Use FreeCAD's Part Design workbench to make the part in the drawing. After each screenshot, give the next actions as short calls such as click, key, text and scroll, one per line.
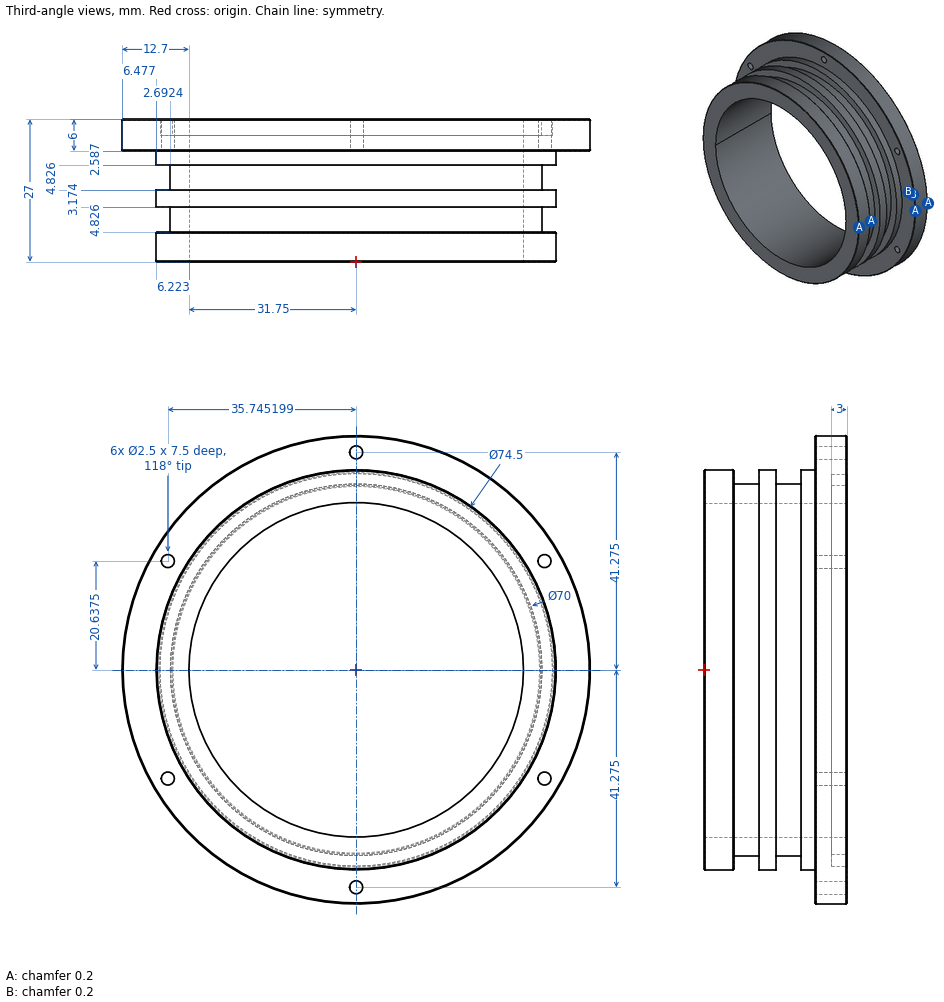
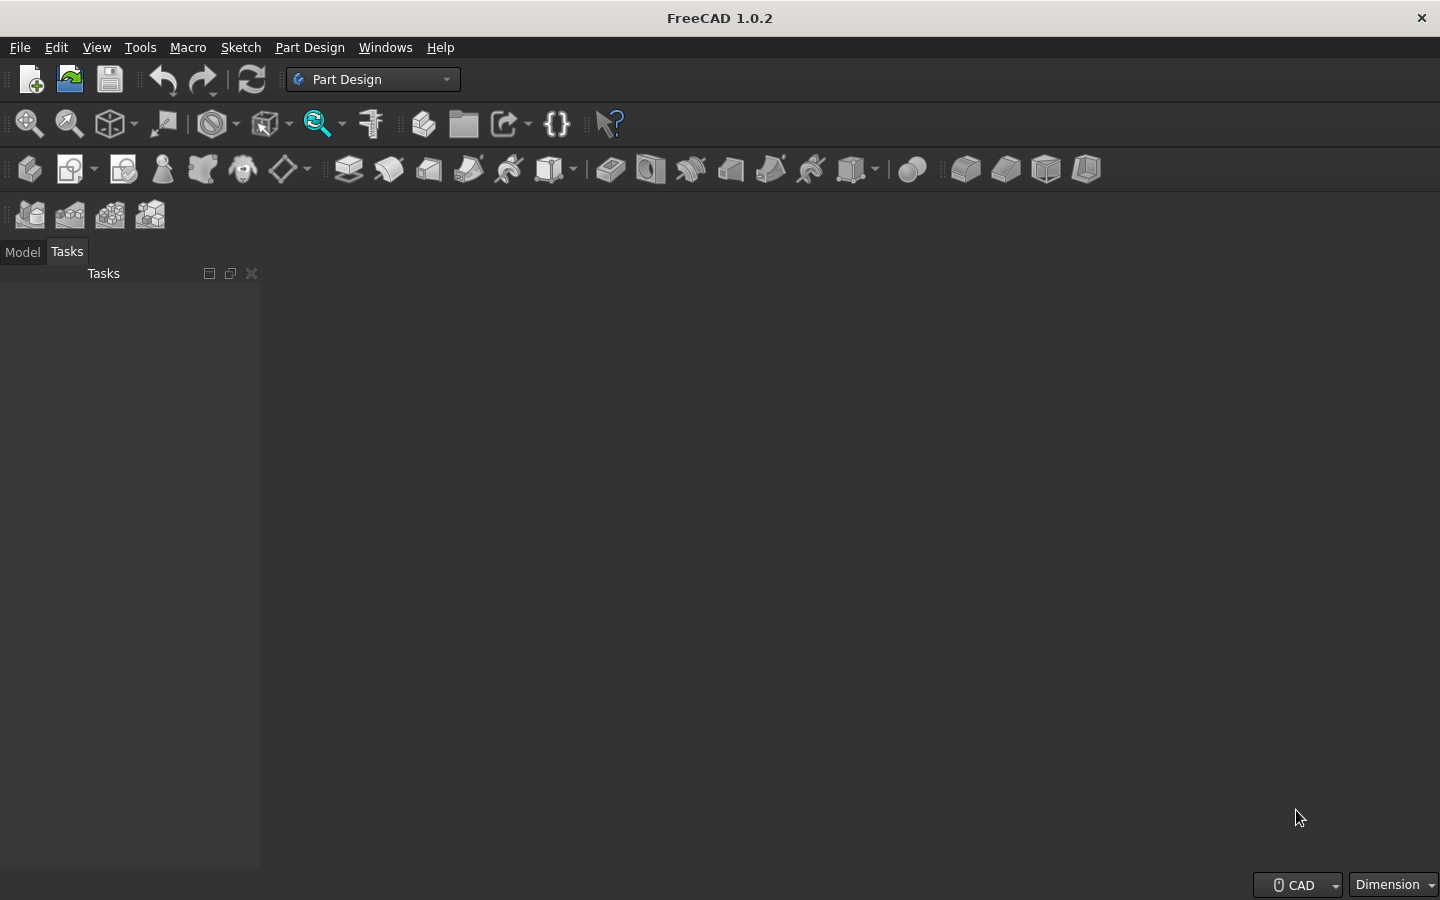
click(30, 80)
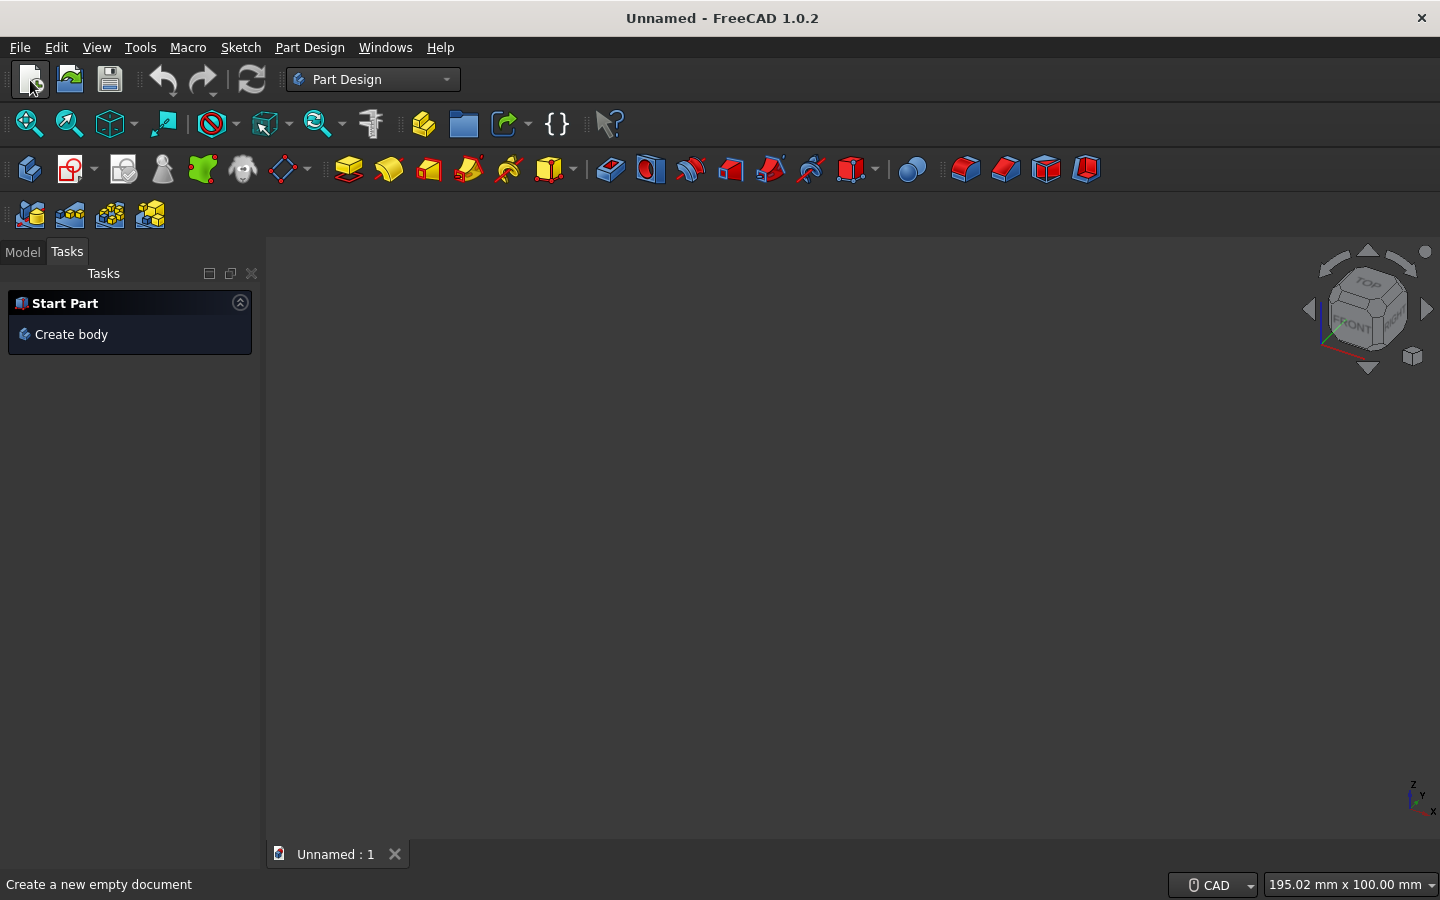
click(70, 170)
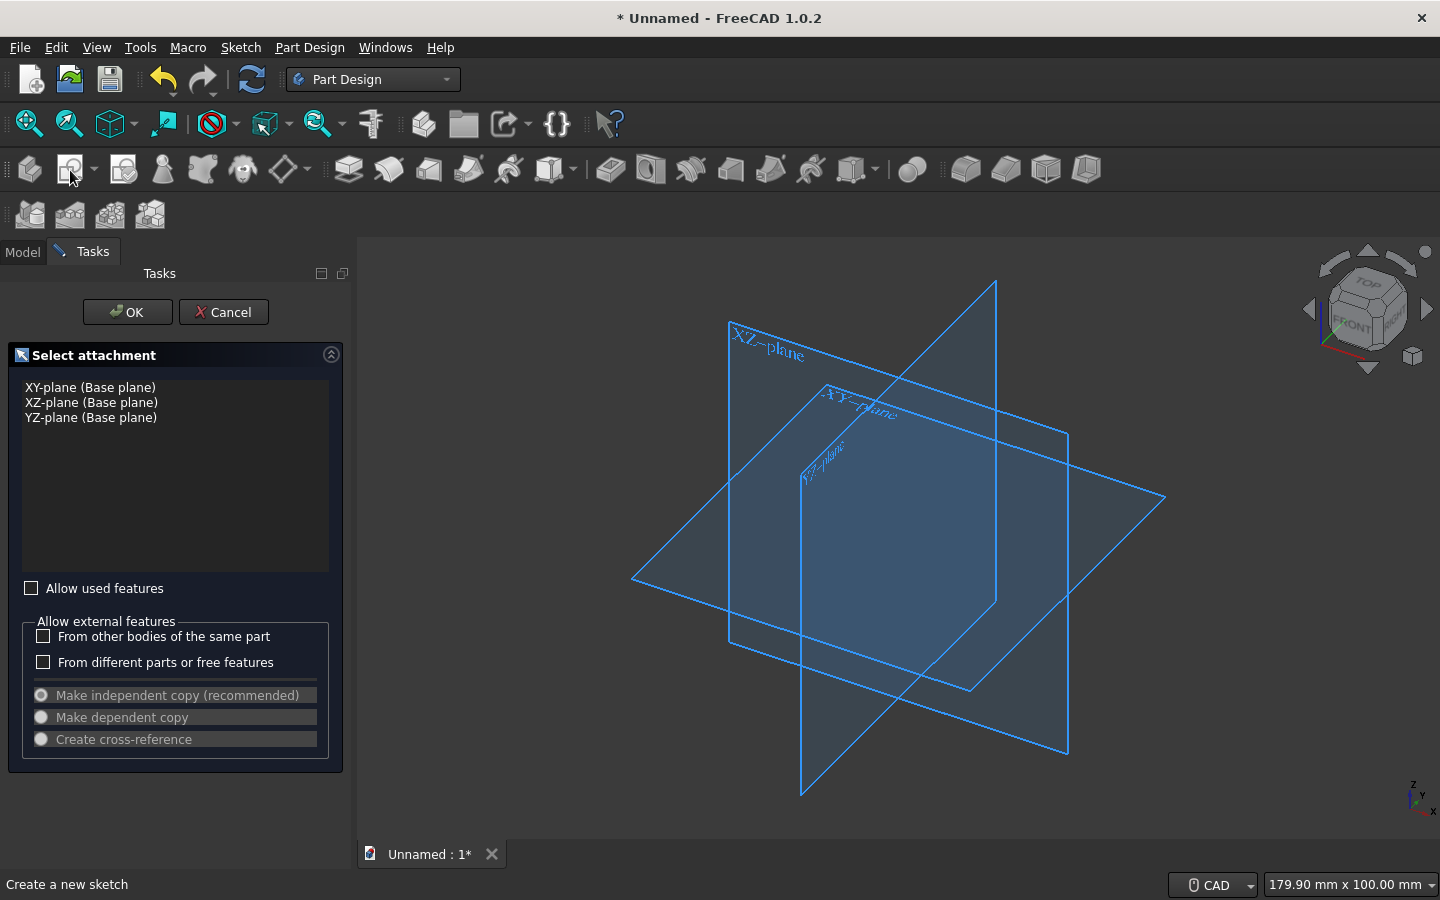
click(82, 388)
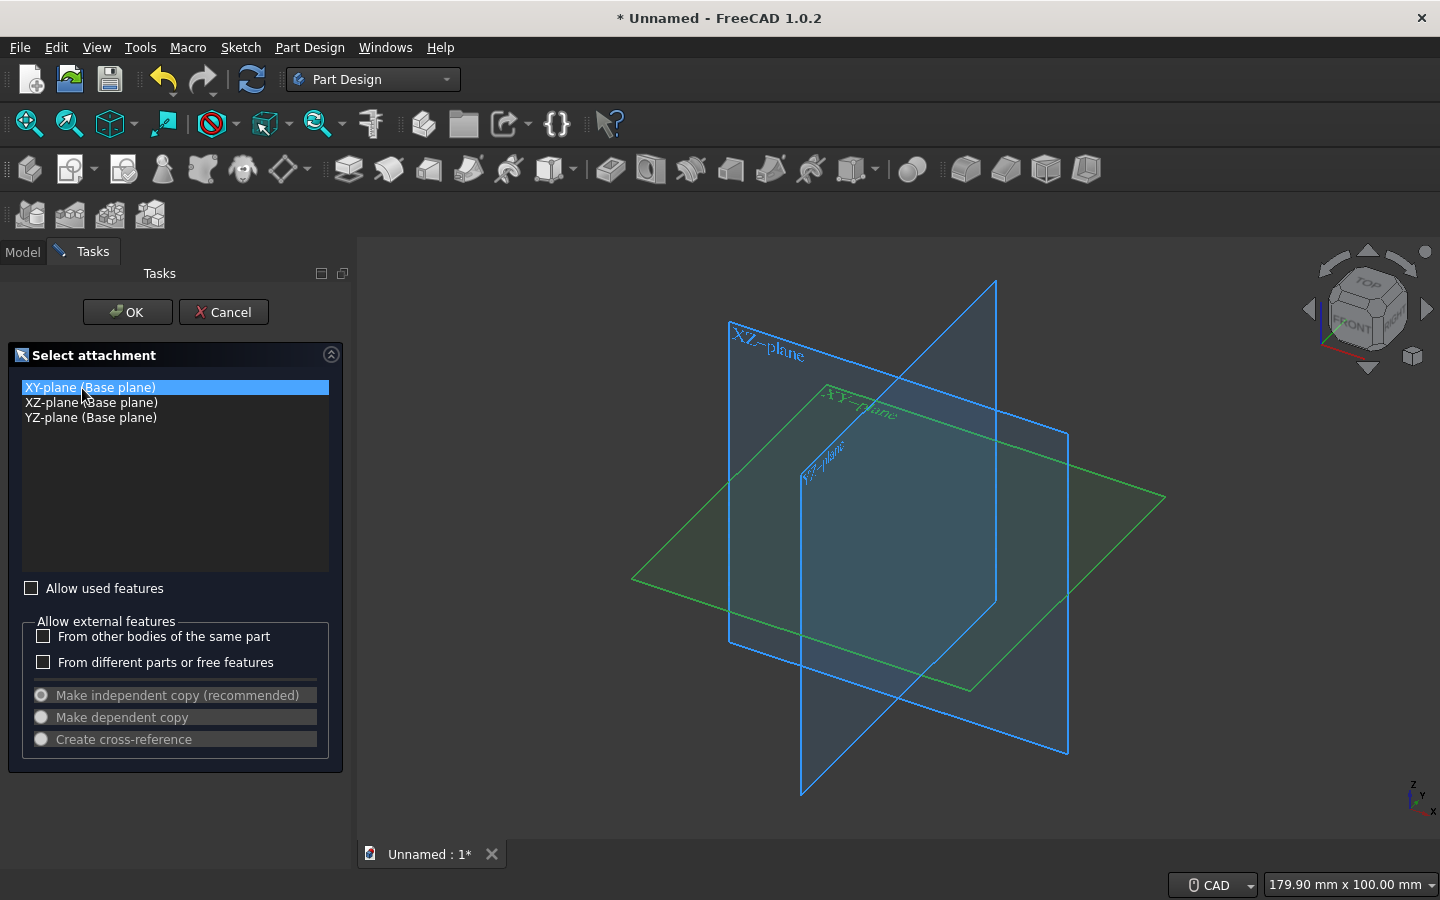
click(128, 312)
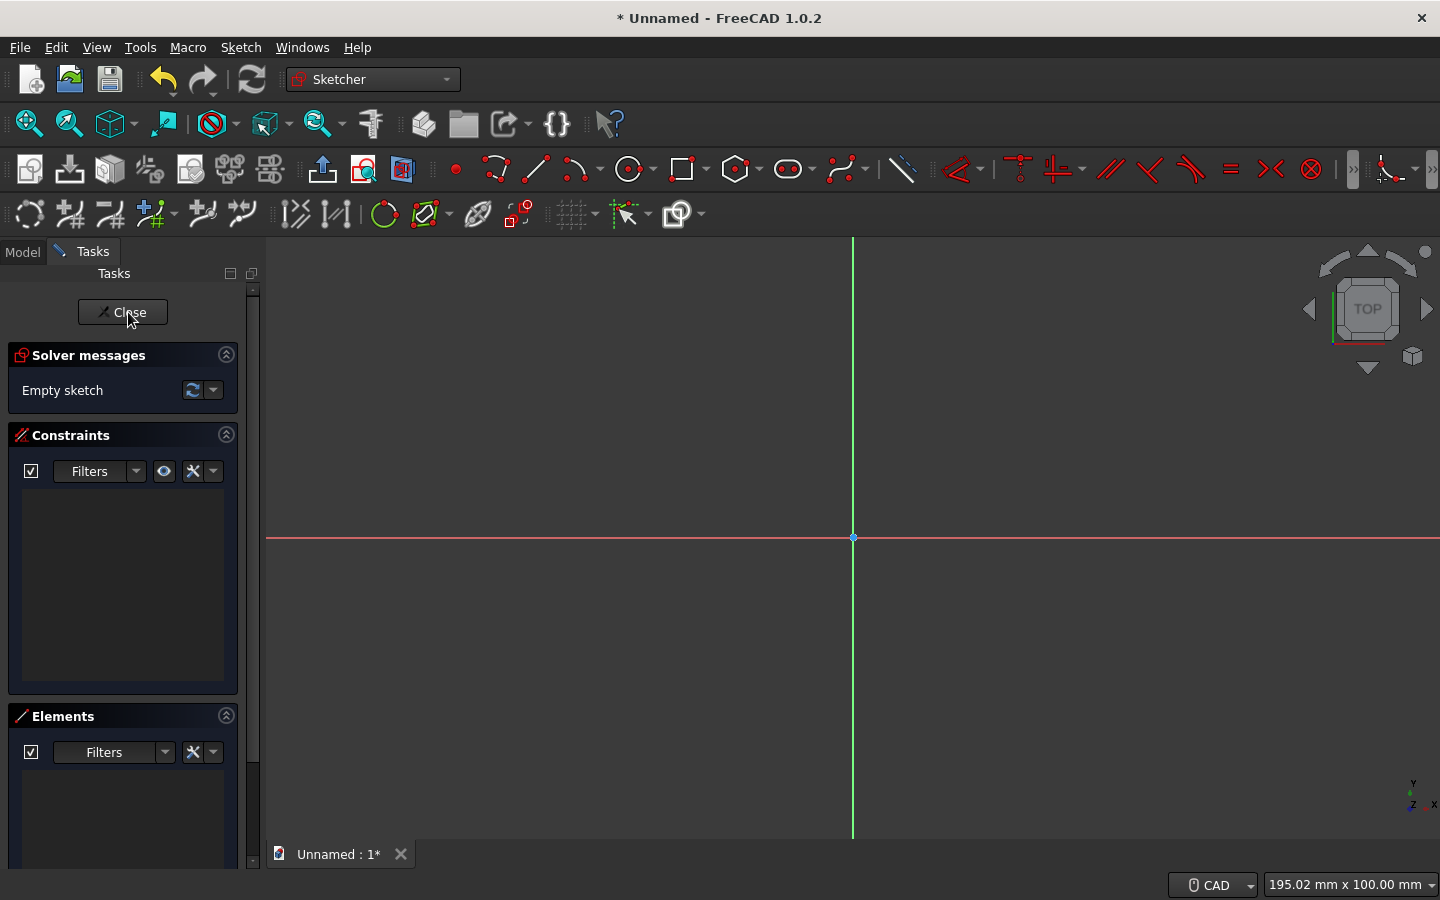
scroll(666, 390, up, 4)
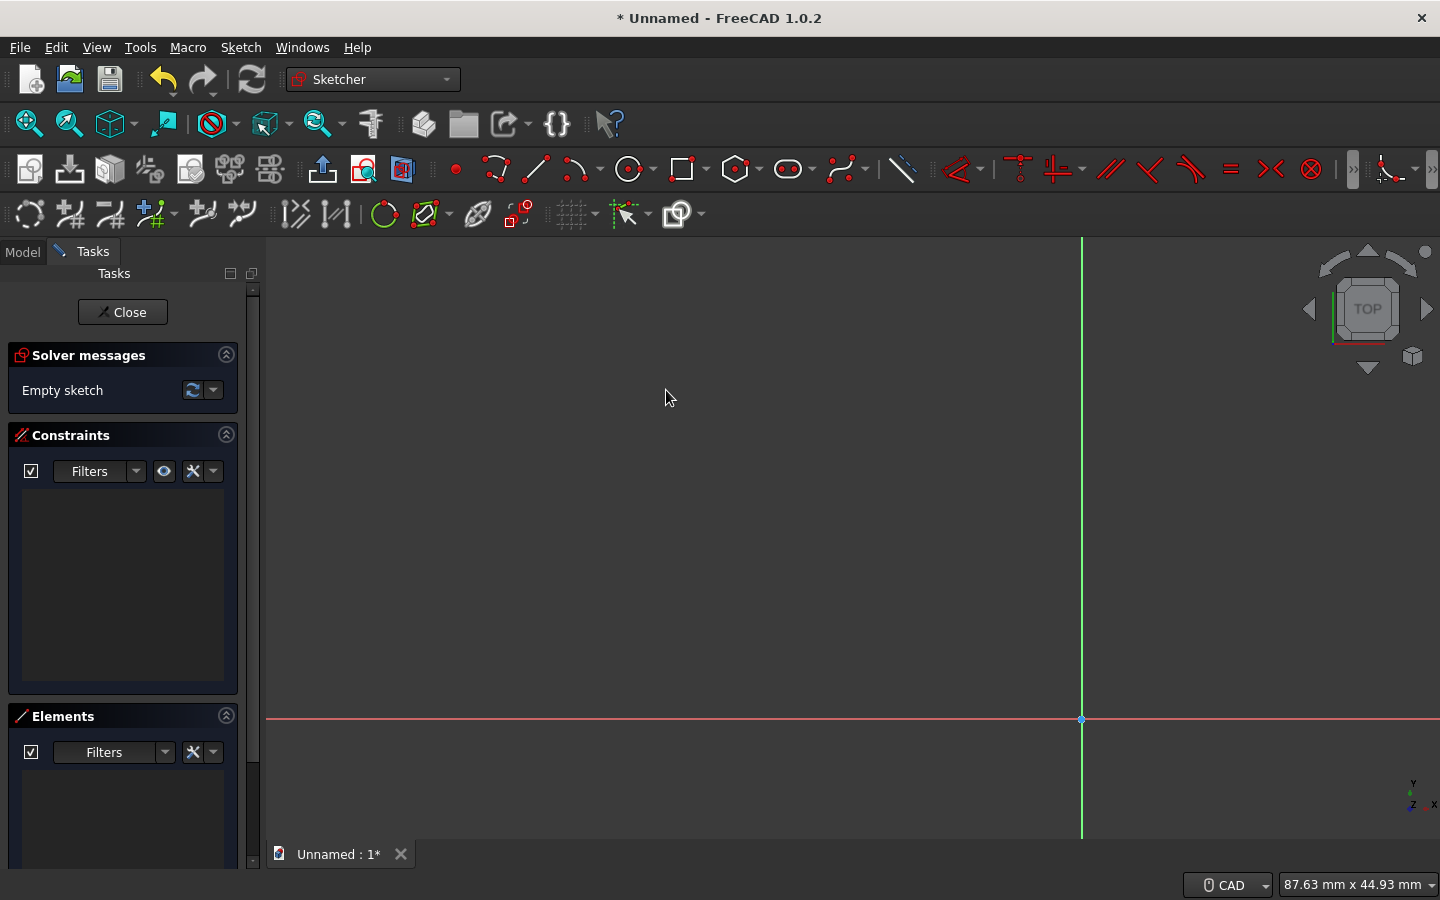
key(g)
key(m)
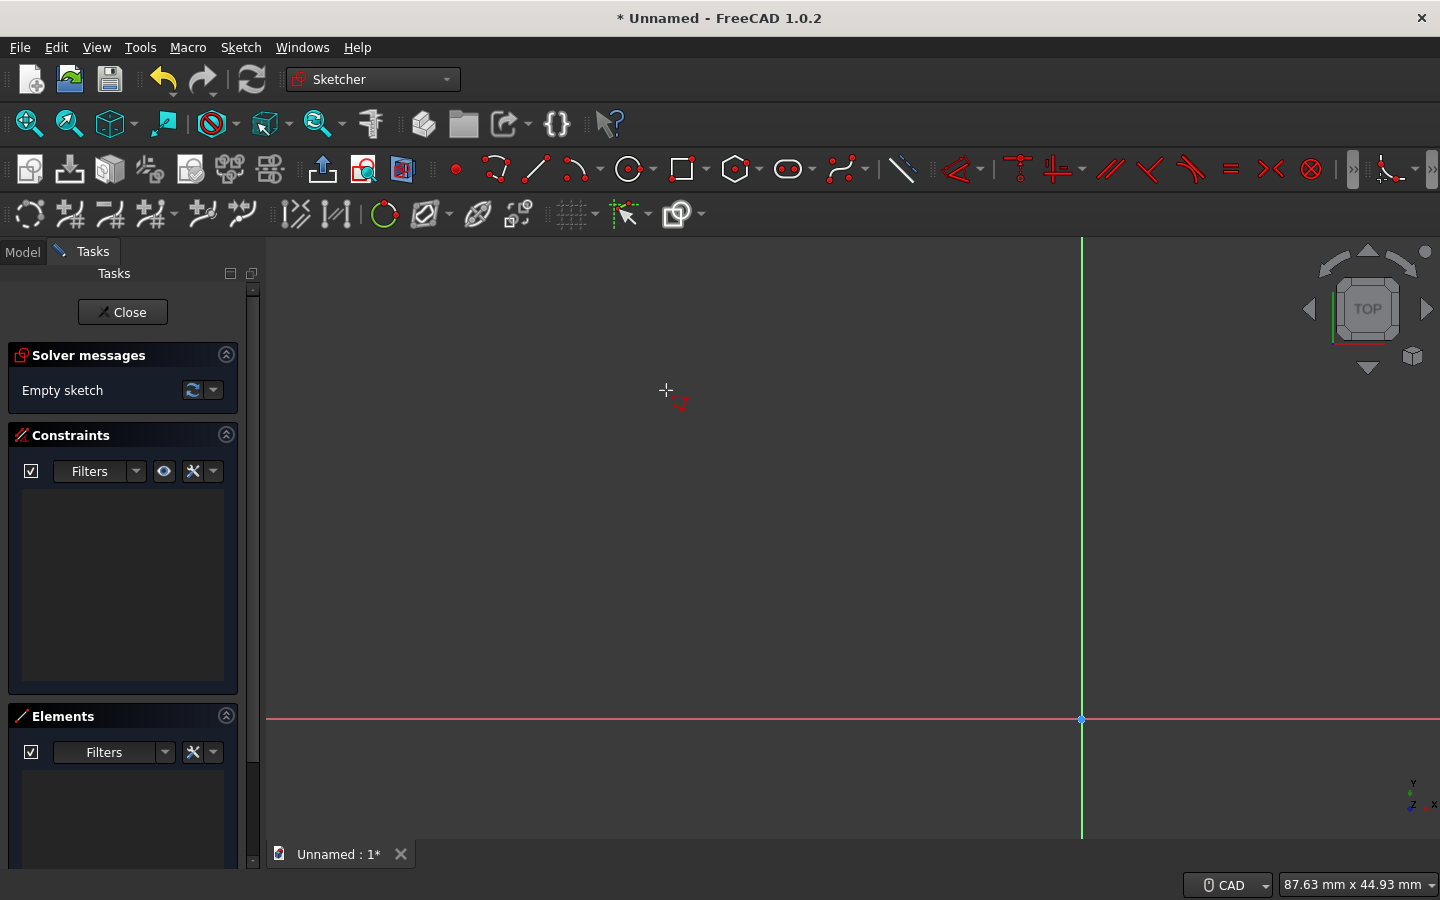
click(656, 719)
click(656, 357)
click(486, 357)
click(486, 438)
click(573, 438)
click(573, 472)
click(609, 472)
click(609, 537)
click(573, 537)
click(573, 580)
click(609, 580)
click(609, 644)
click(573, 644)
click(573, 710)
click(656, 719)
key(Escape)
key(Escape)